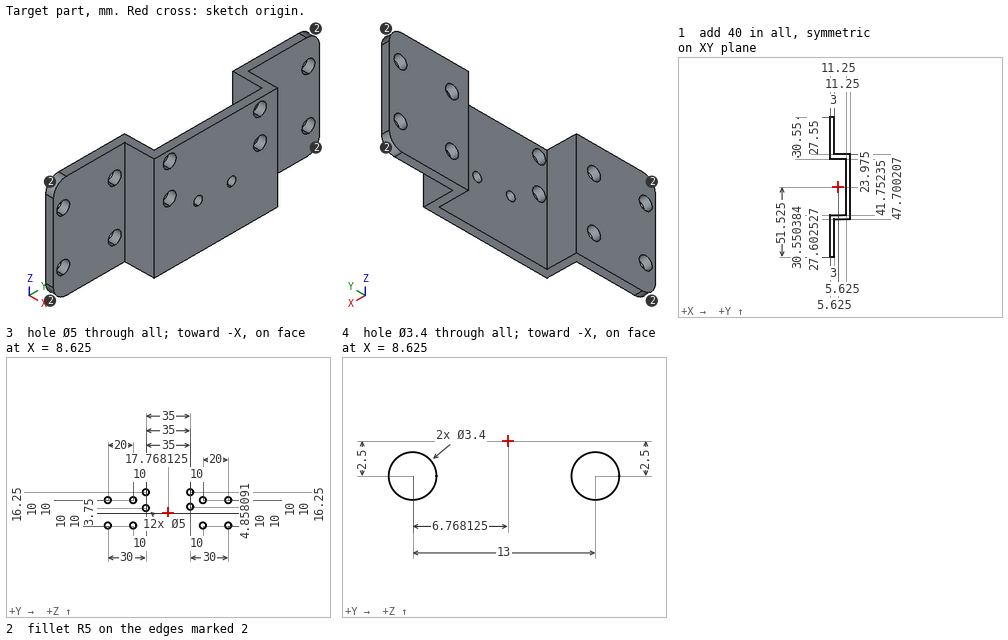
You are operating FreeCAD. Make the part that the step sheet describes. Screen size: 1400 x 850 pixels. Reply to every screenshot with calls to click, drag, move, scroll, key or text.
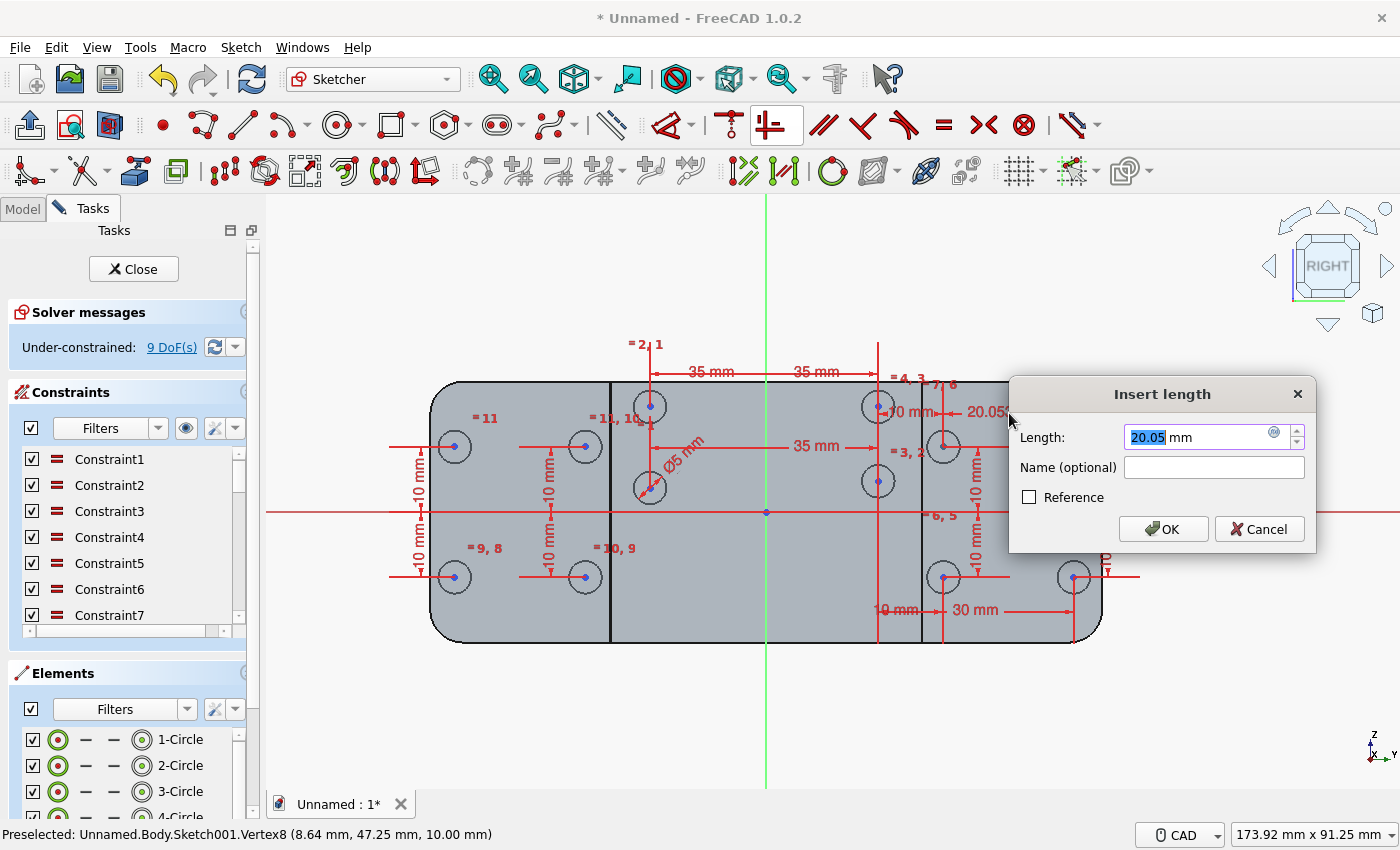
text(20)
key(Return)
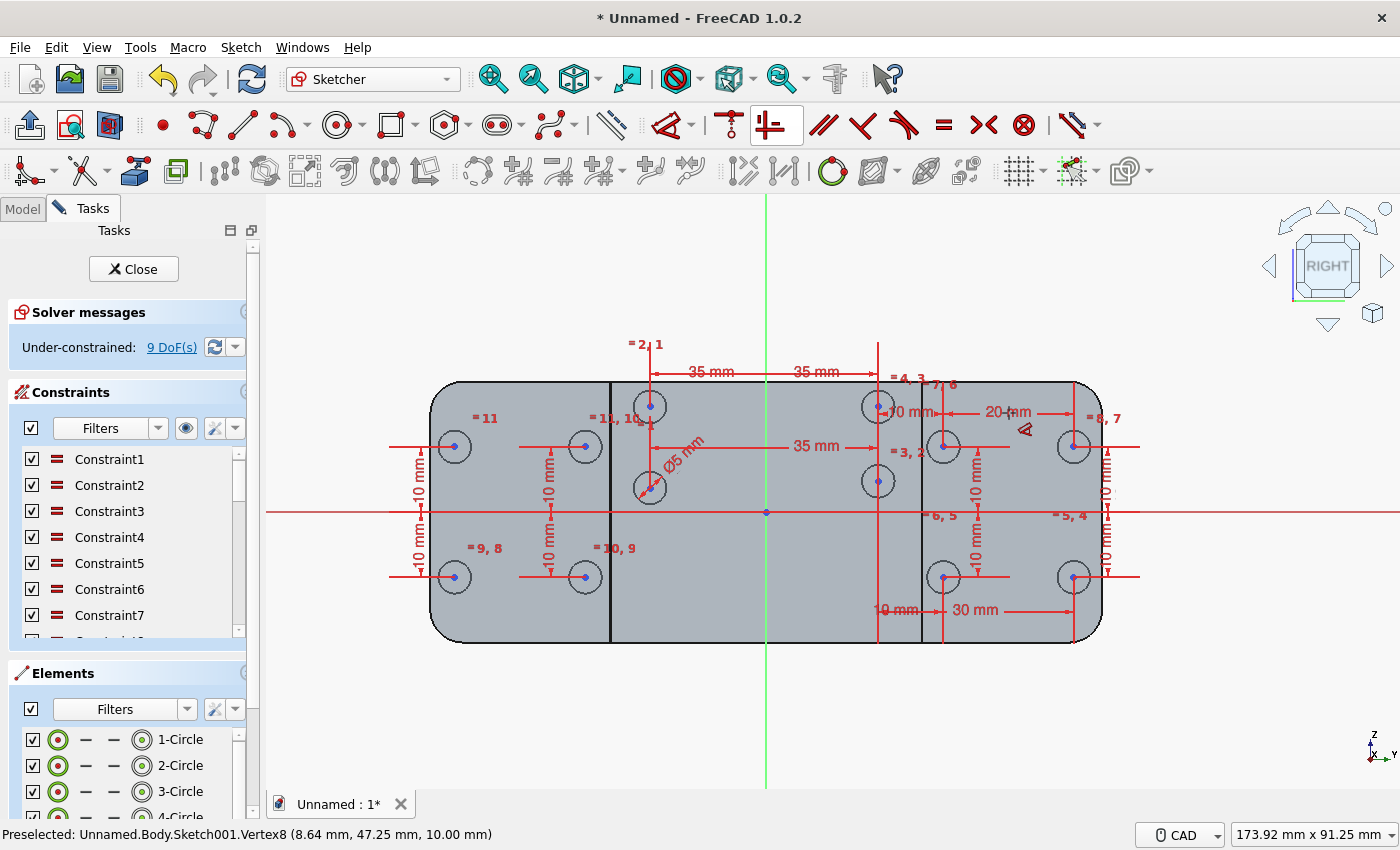
click(650, 488)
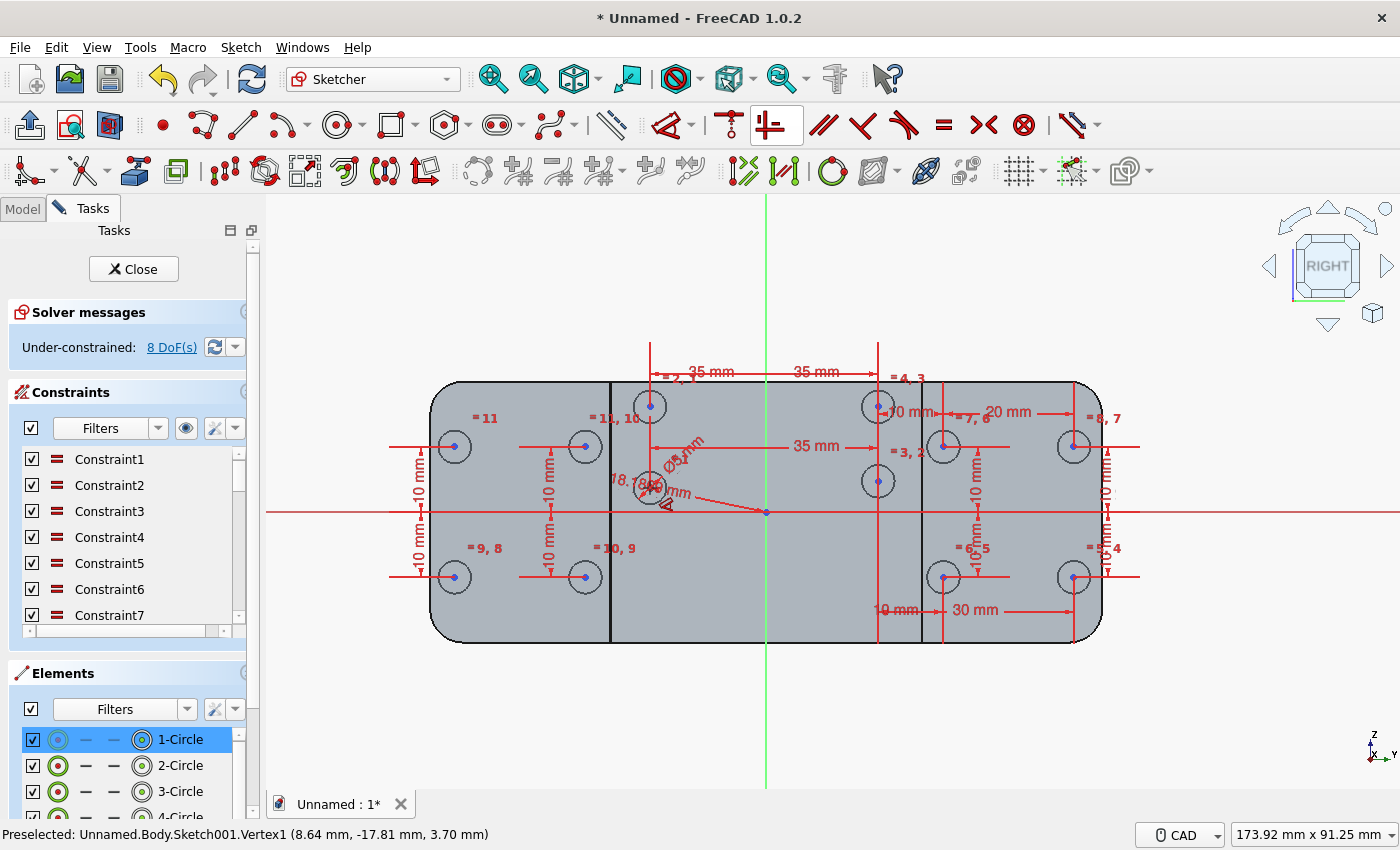
click(455, 577)
click(552, 611)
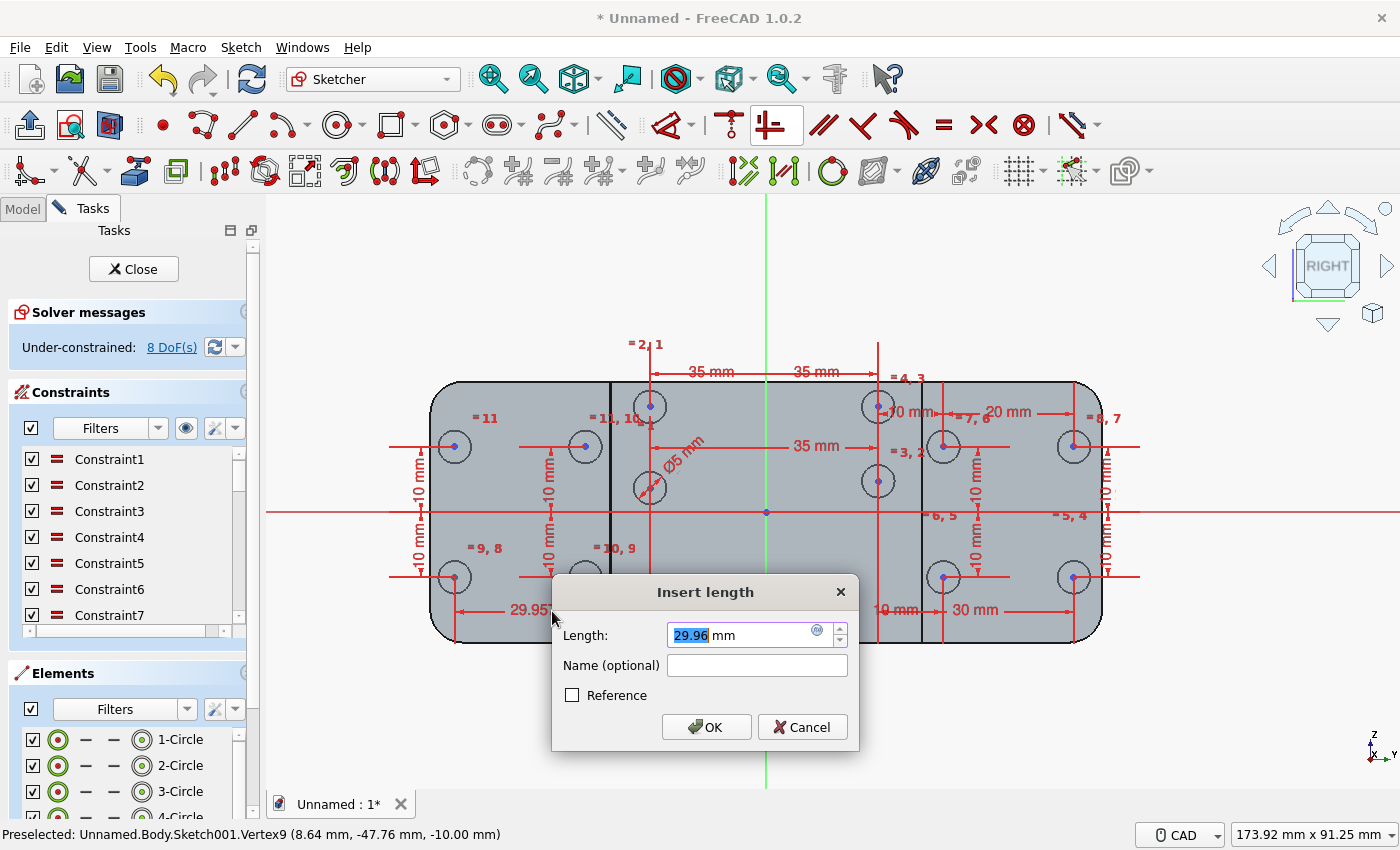
text(30)
key(Return)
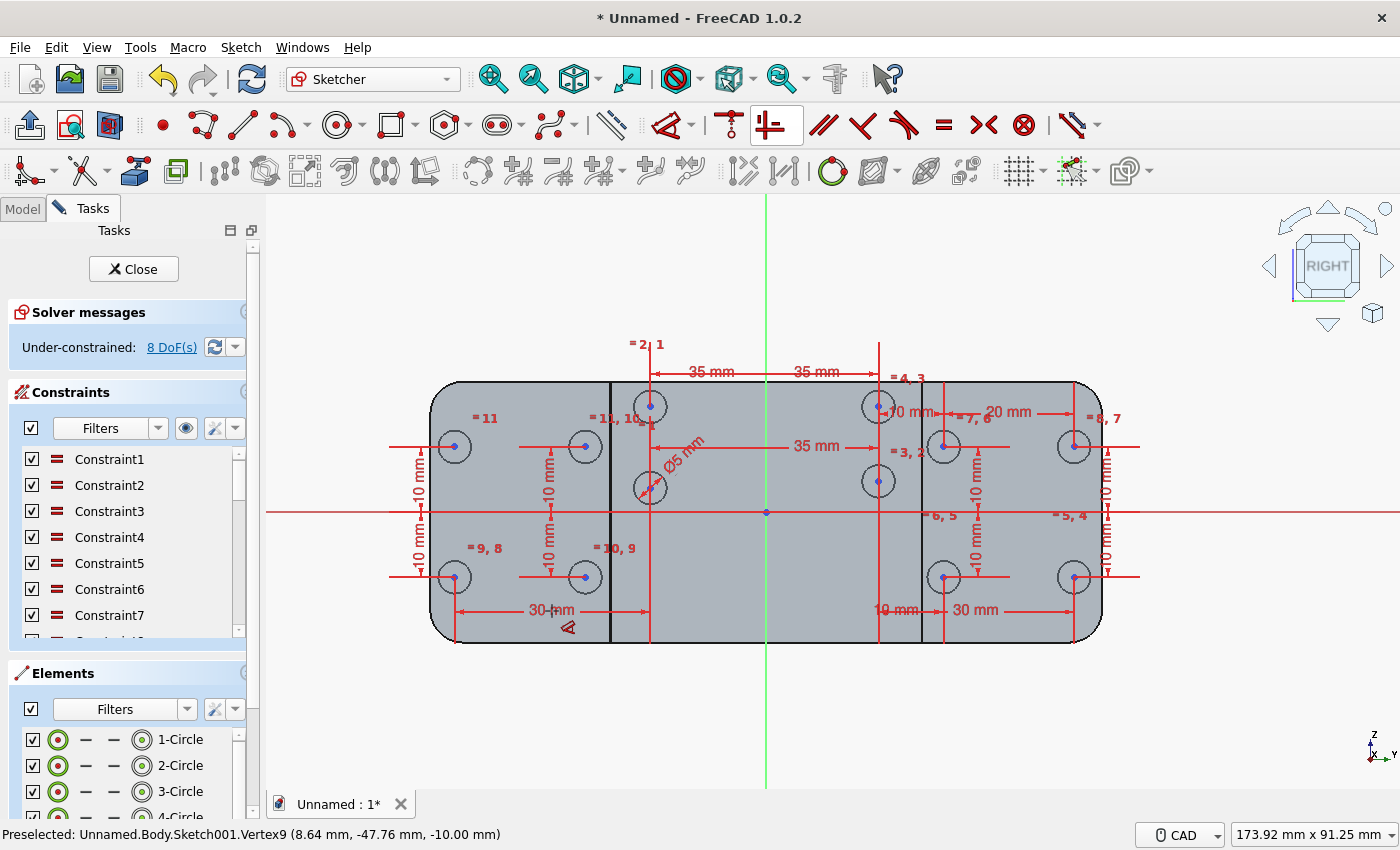
click(650, 488)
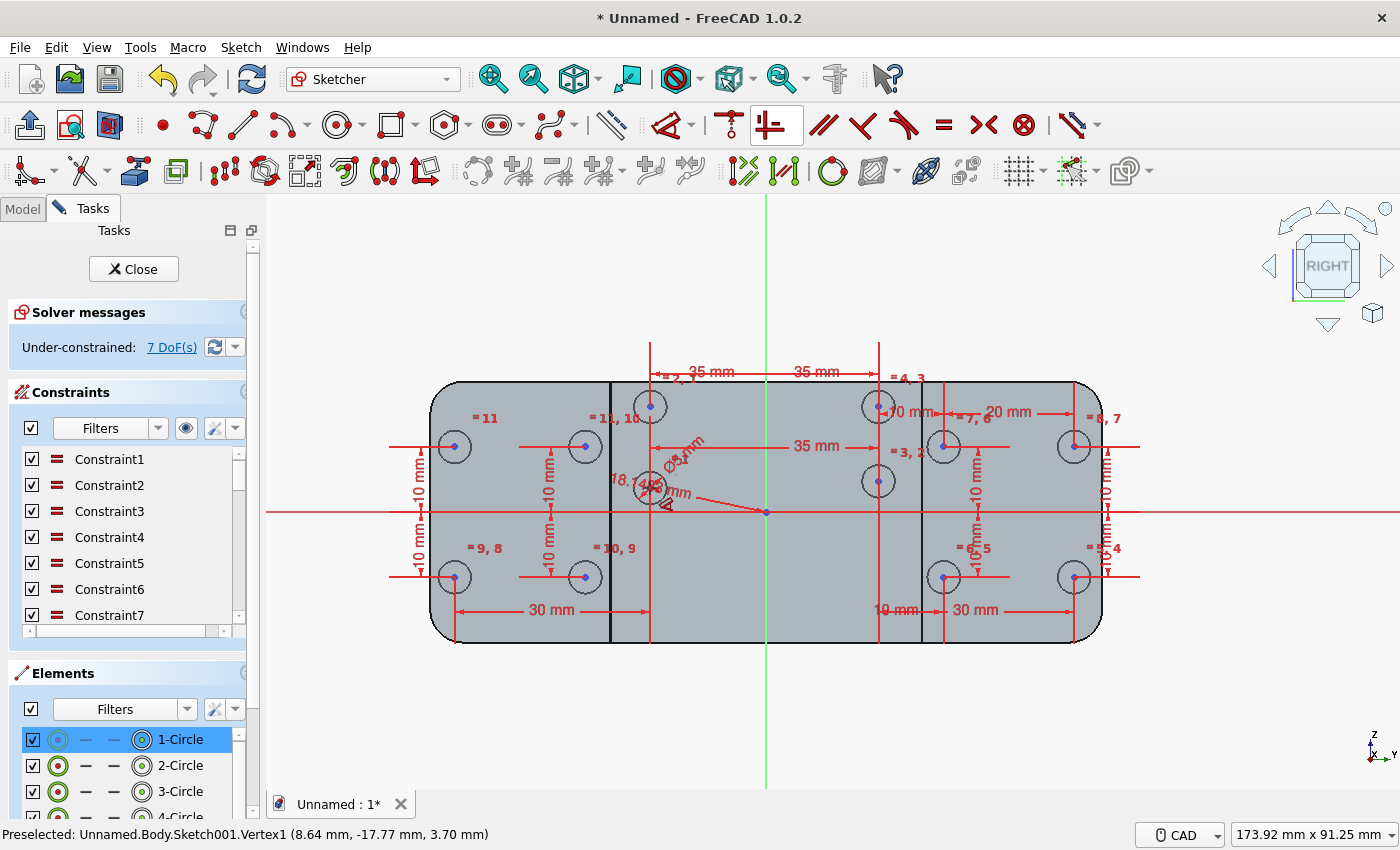
click(585, 577)
click(633, 611)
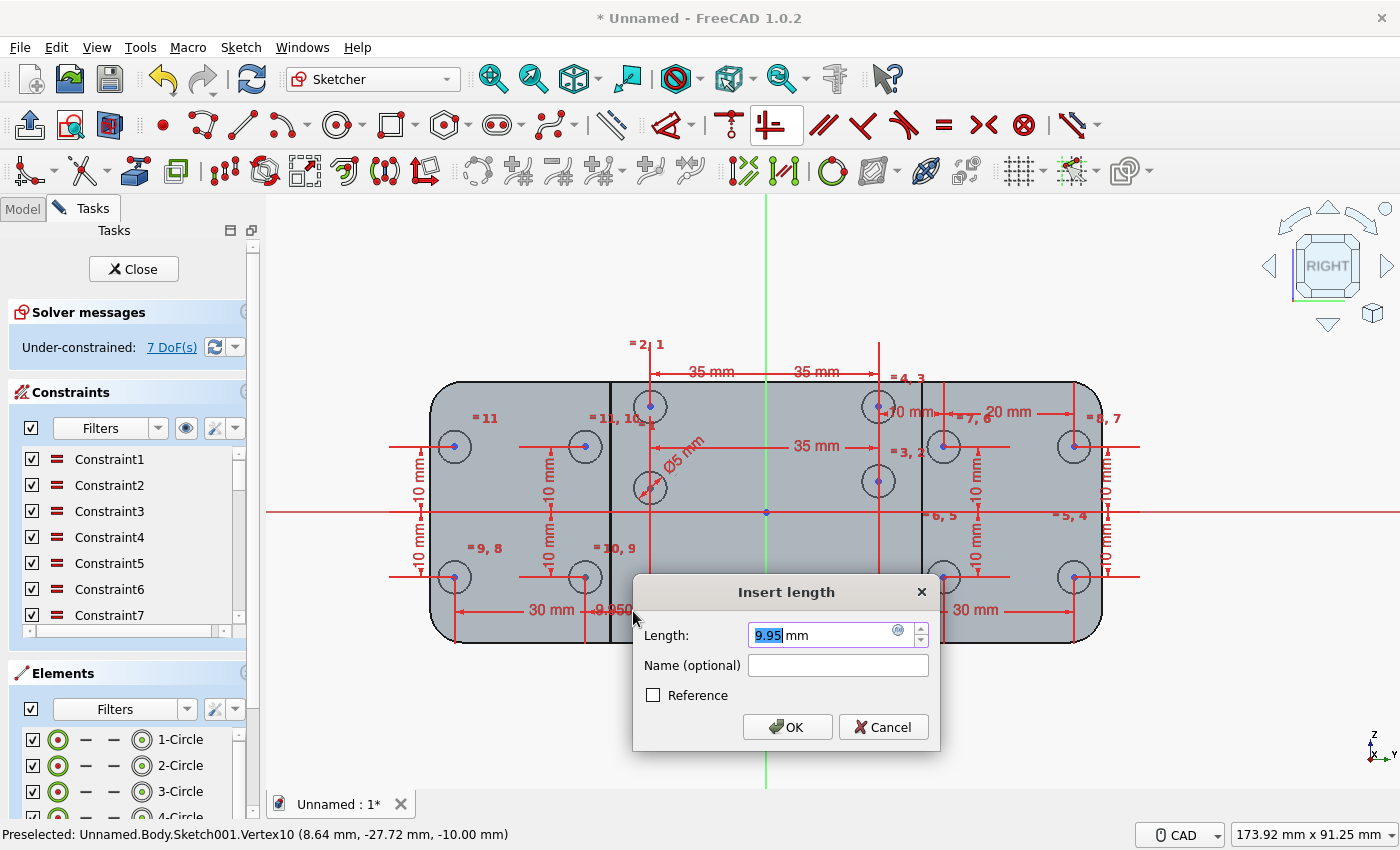
text(10)
key(Return)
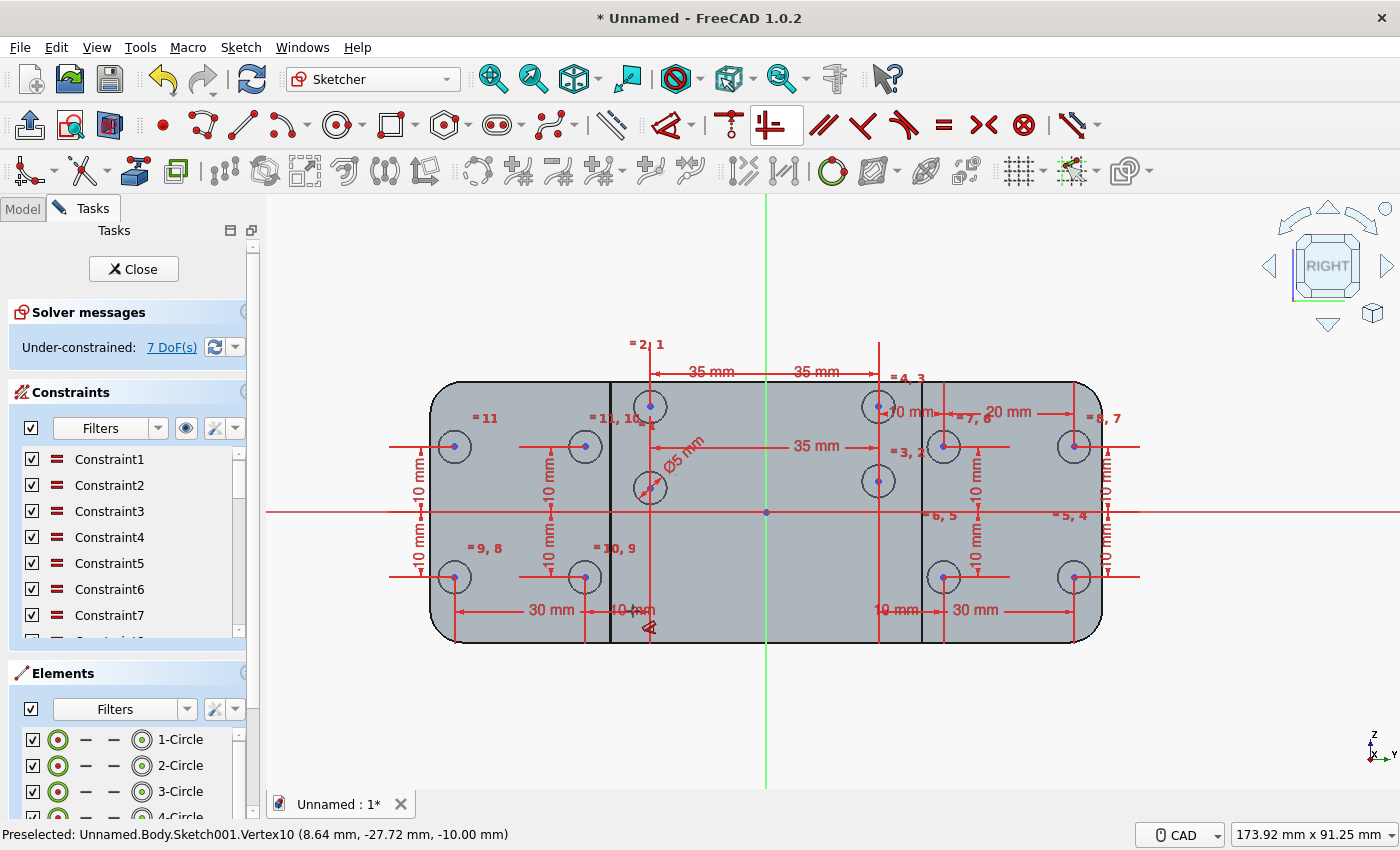
click(650, 488)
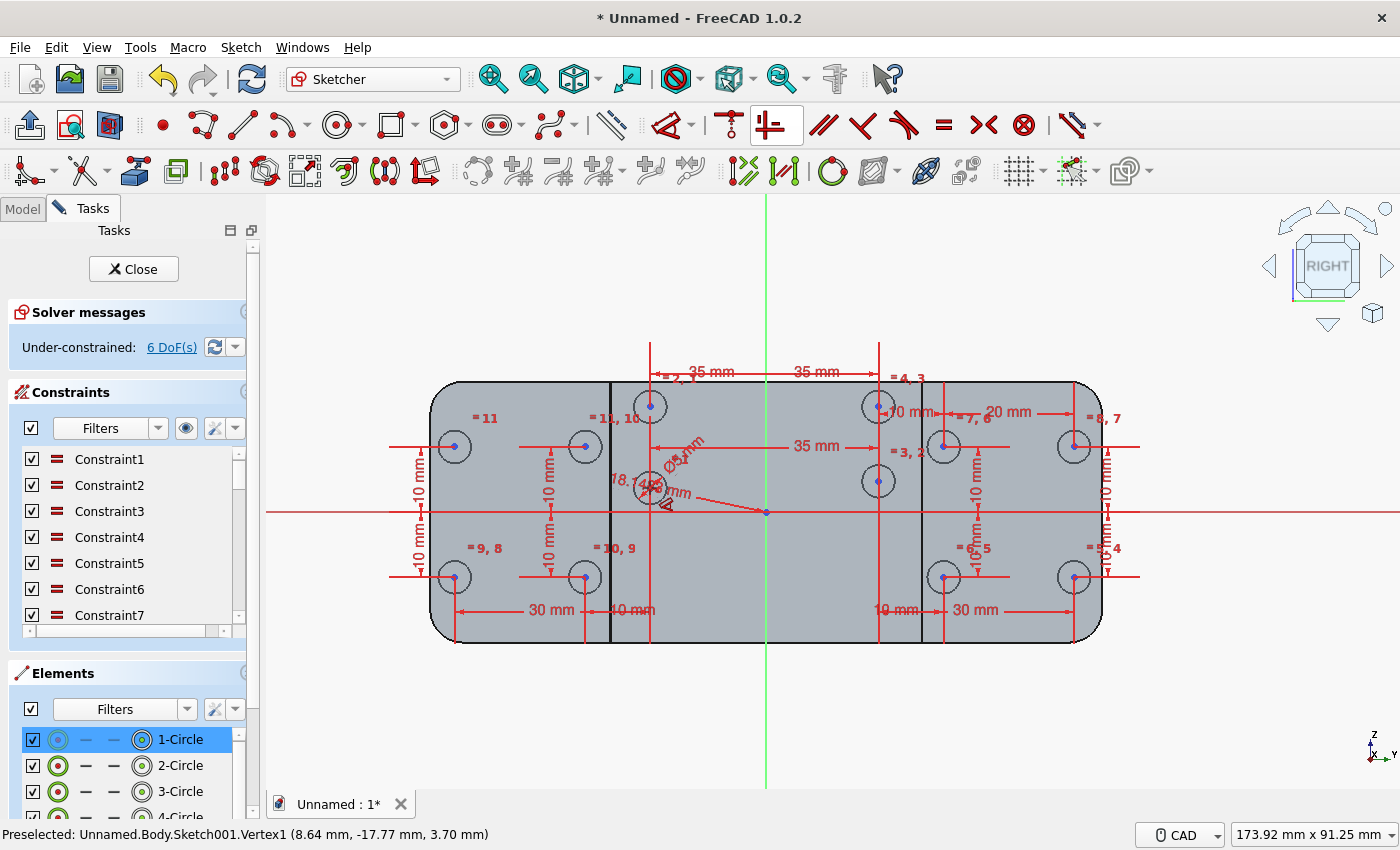
click(585, 447)
click(618, 413)